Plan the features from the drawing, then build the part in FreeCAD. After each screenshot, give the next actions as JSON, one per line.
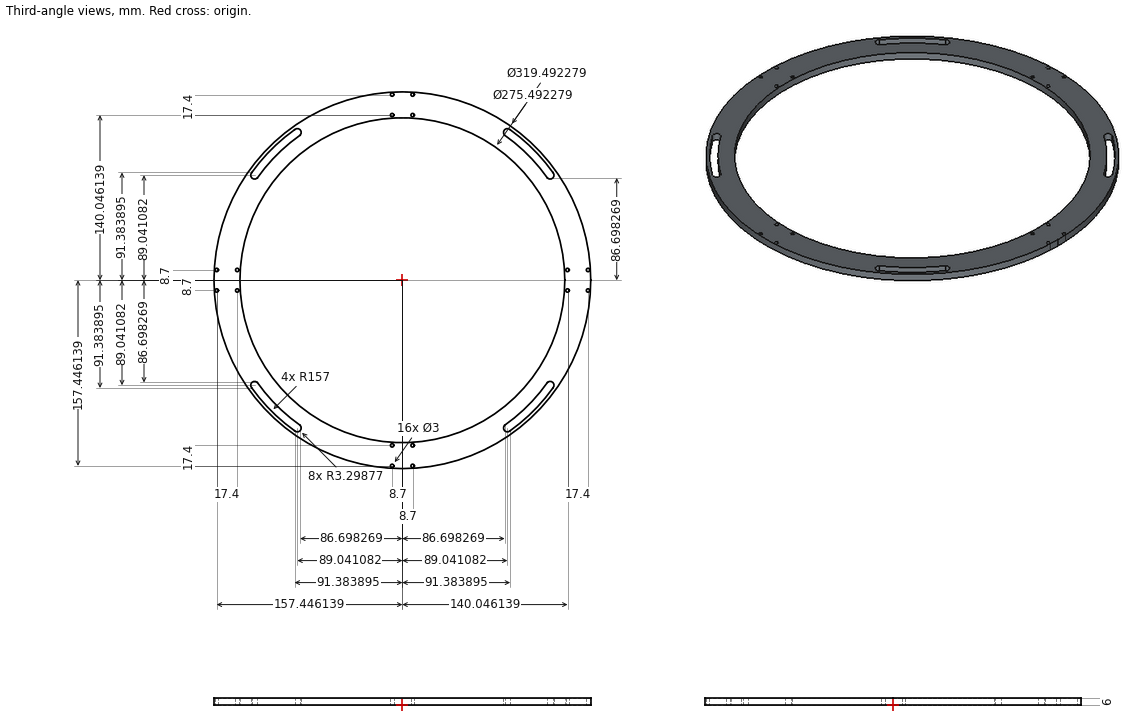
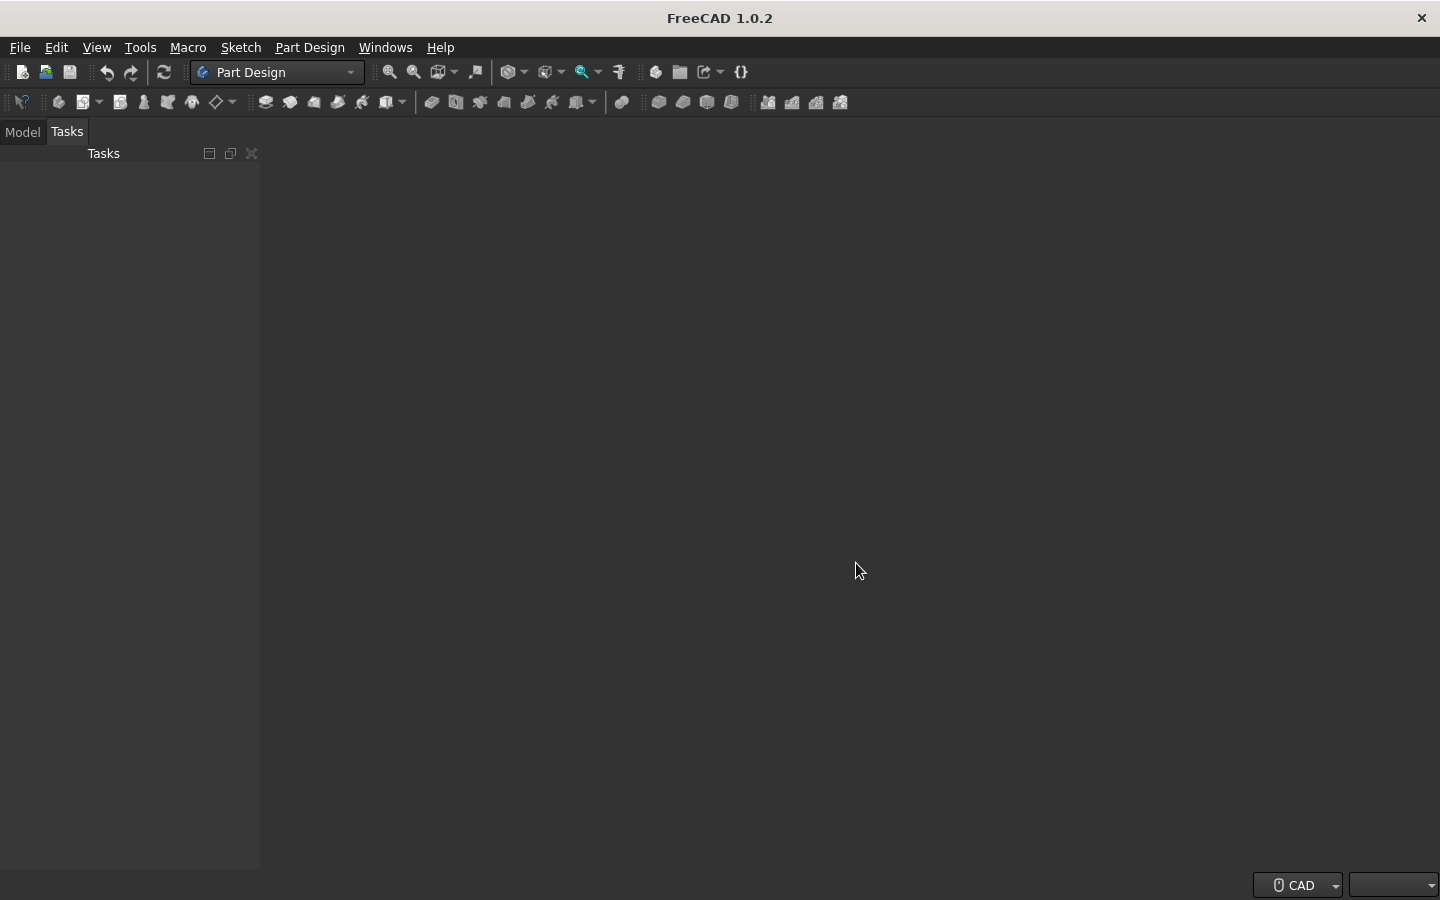
{"action": "key", "text": "ctrl+n"}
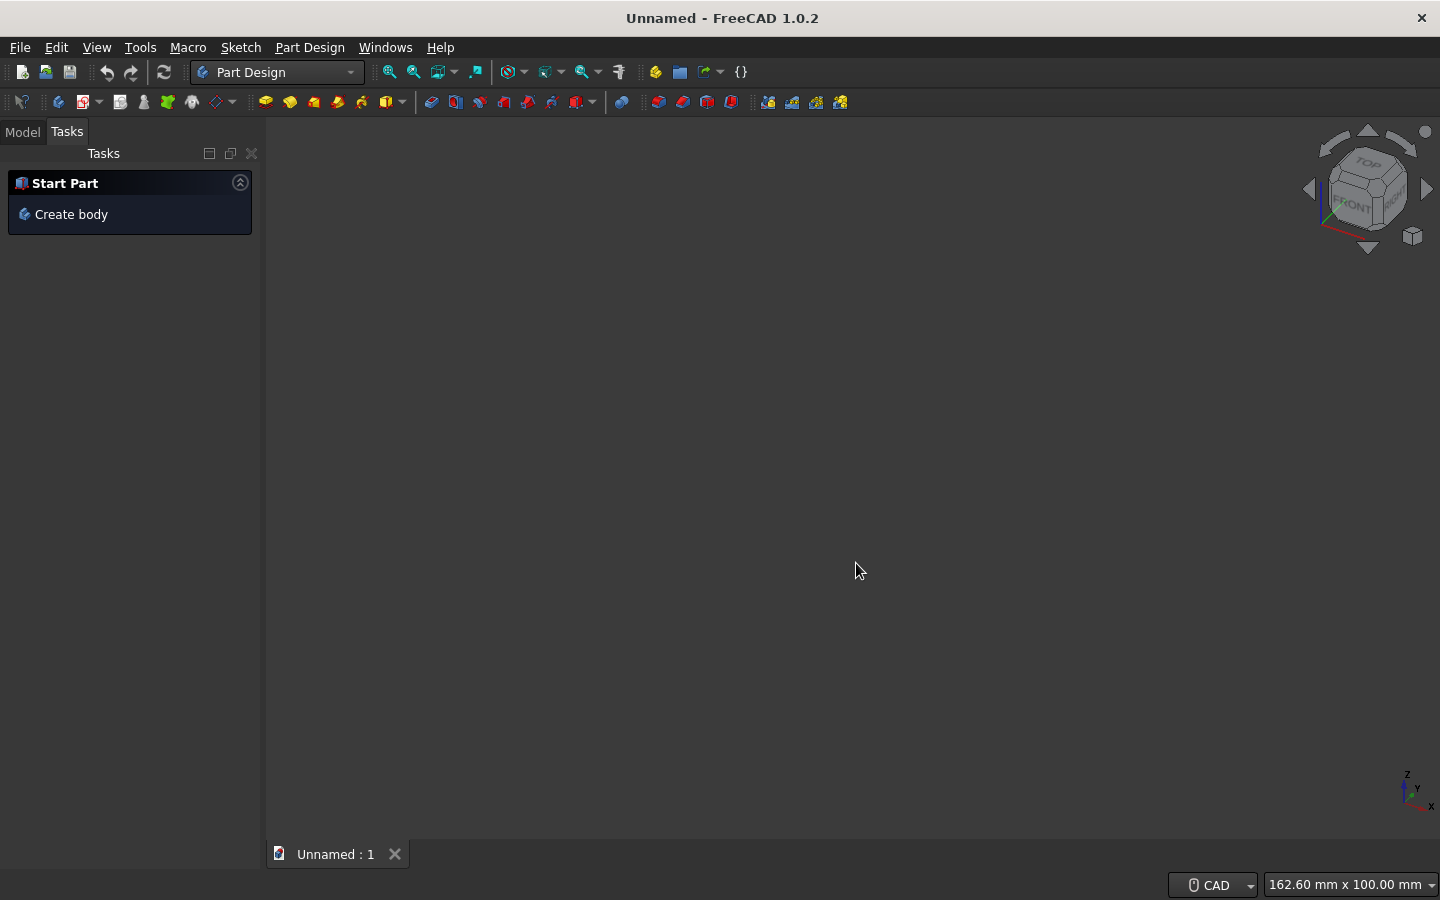
{"action": "left_click", "coordinate": [84, 102]}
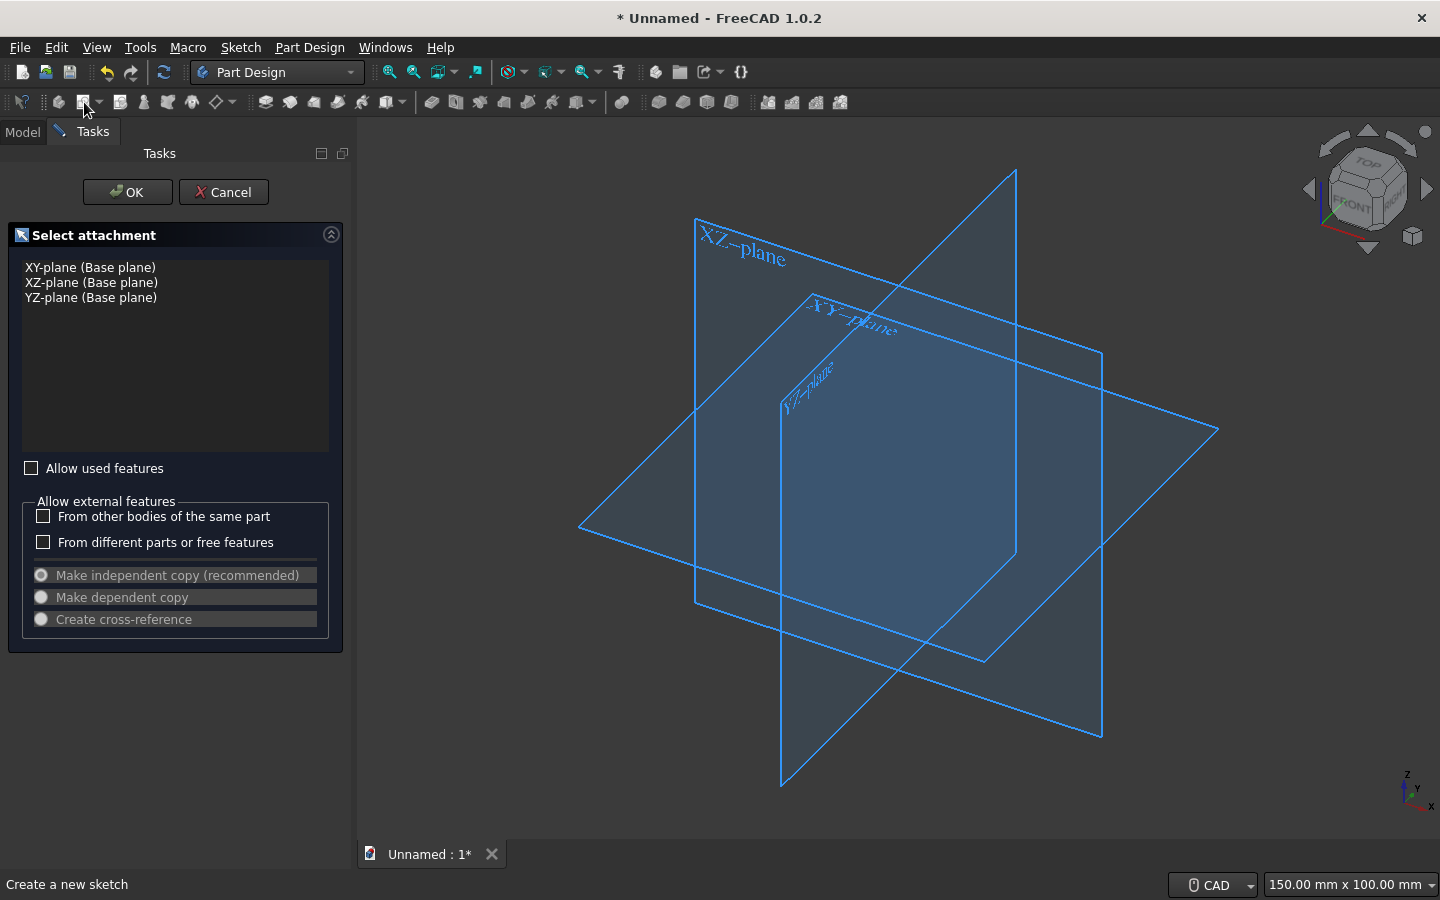
{"action": "left_click", "coordinate": [82, 268]}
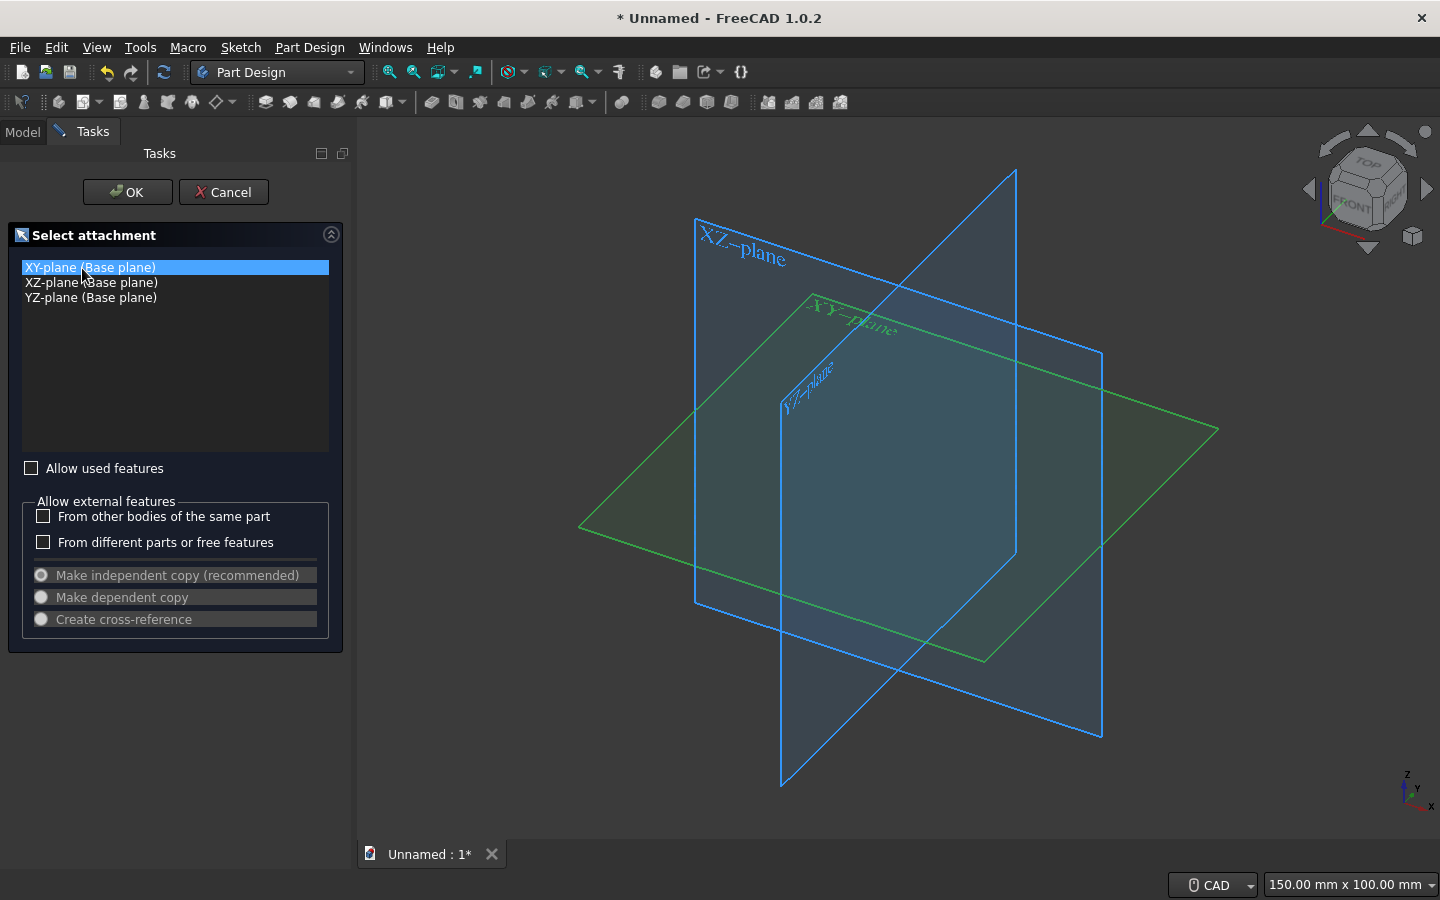
{"action": "left_click", "coordinate": [128, 192]}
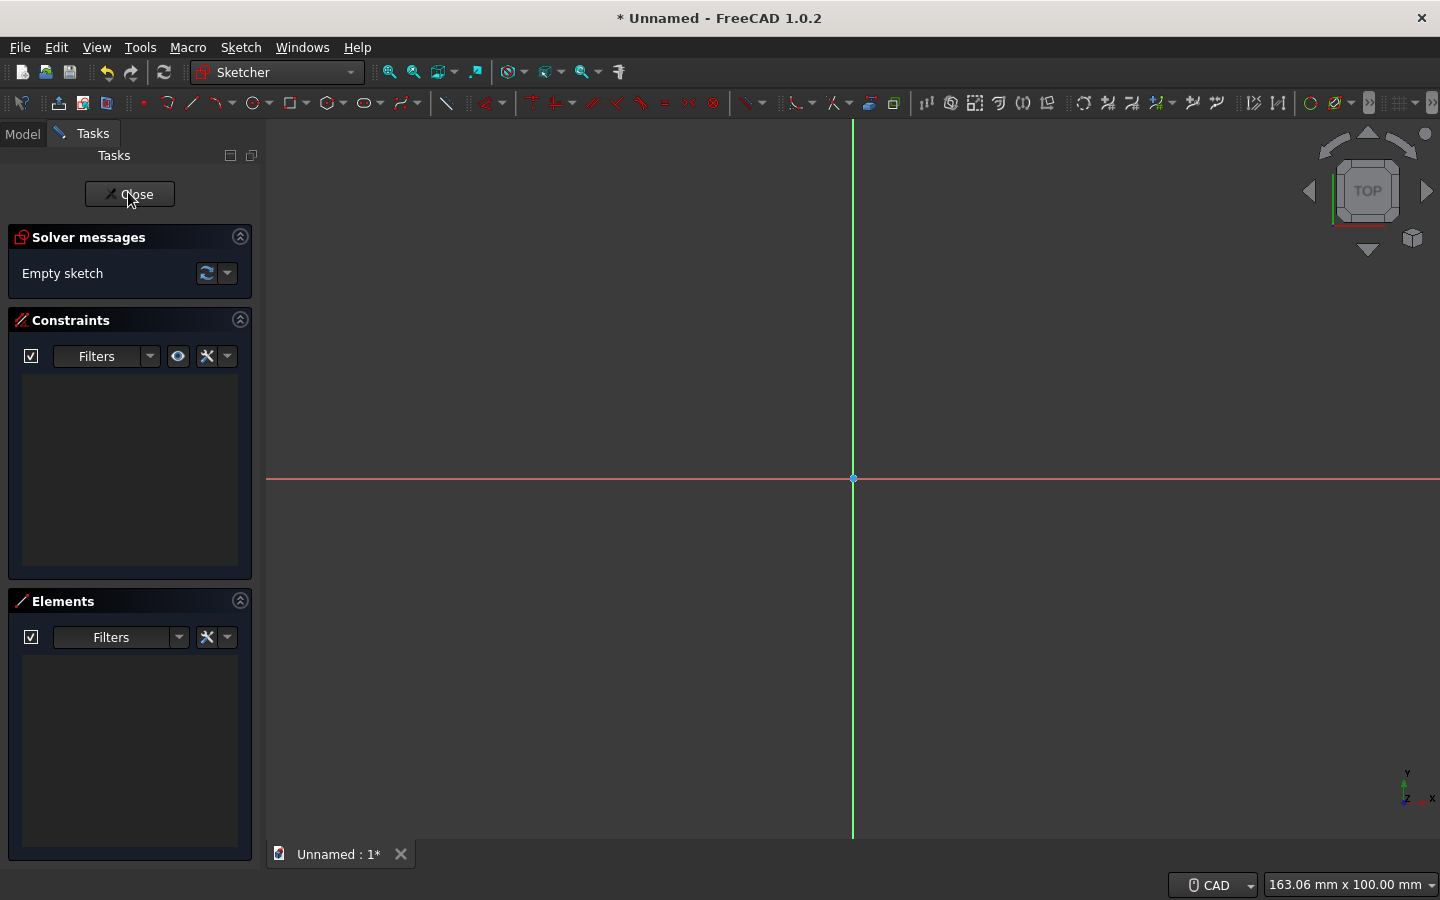
{"action": "scroll", "coordinate": [767, 479], "scroll_direction": "down", "scroll_amount": 8}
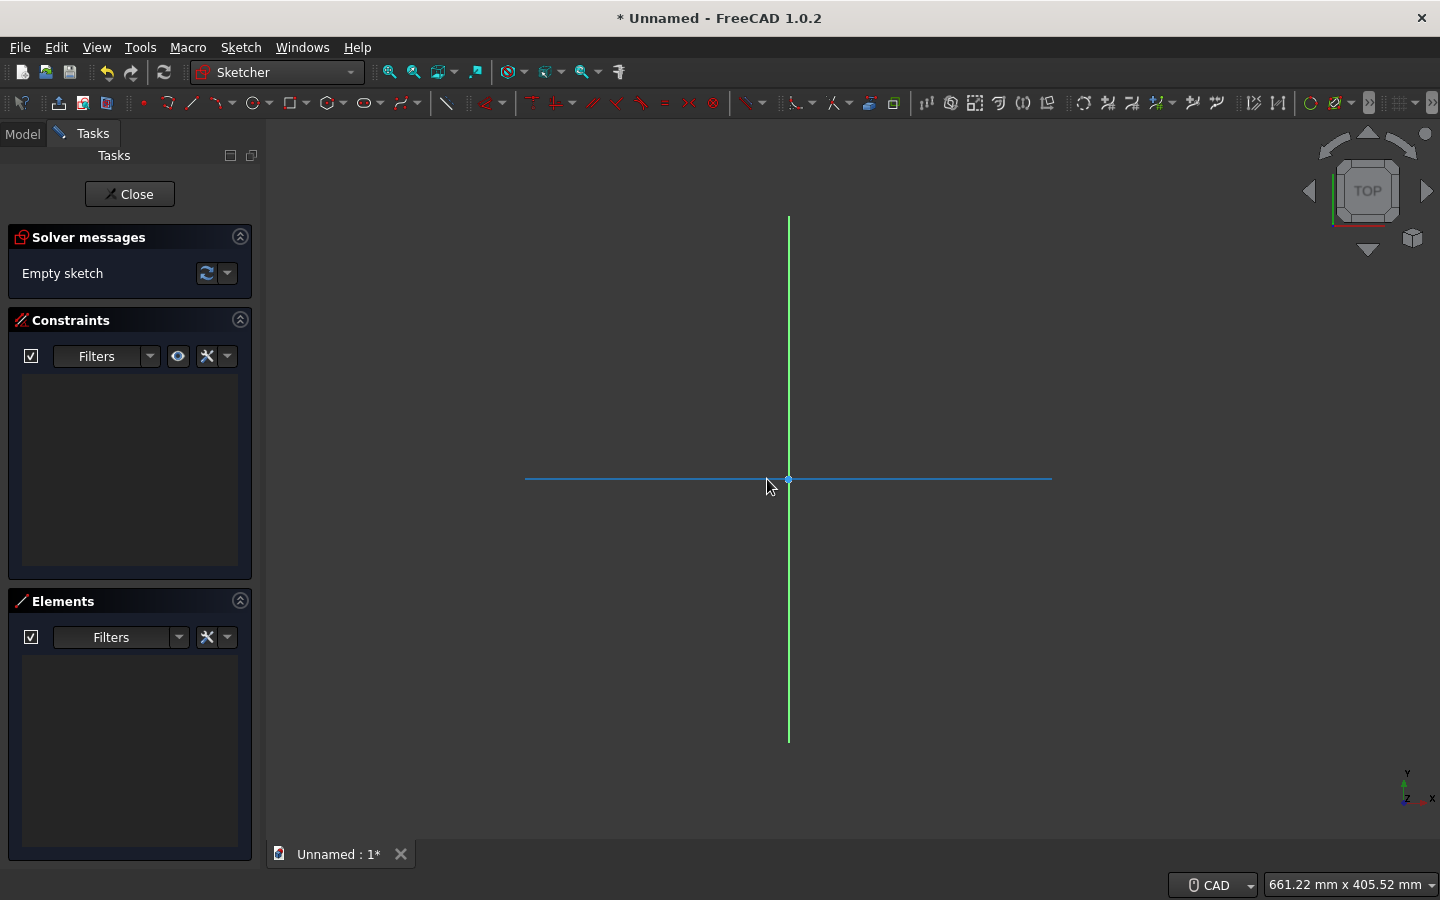
{"action": "key", "text": "g 3 a"}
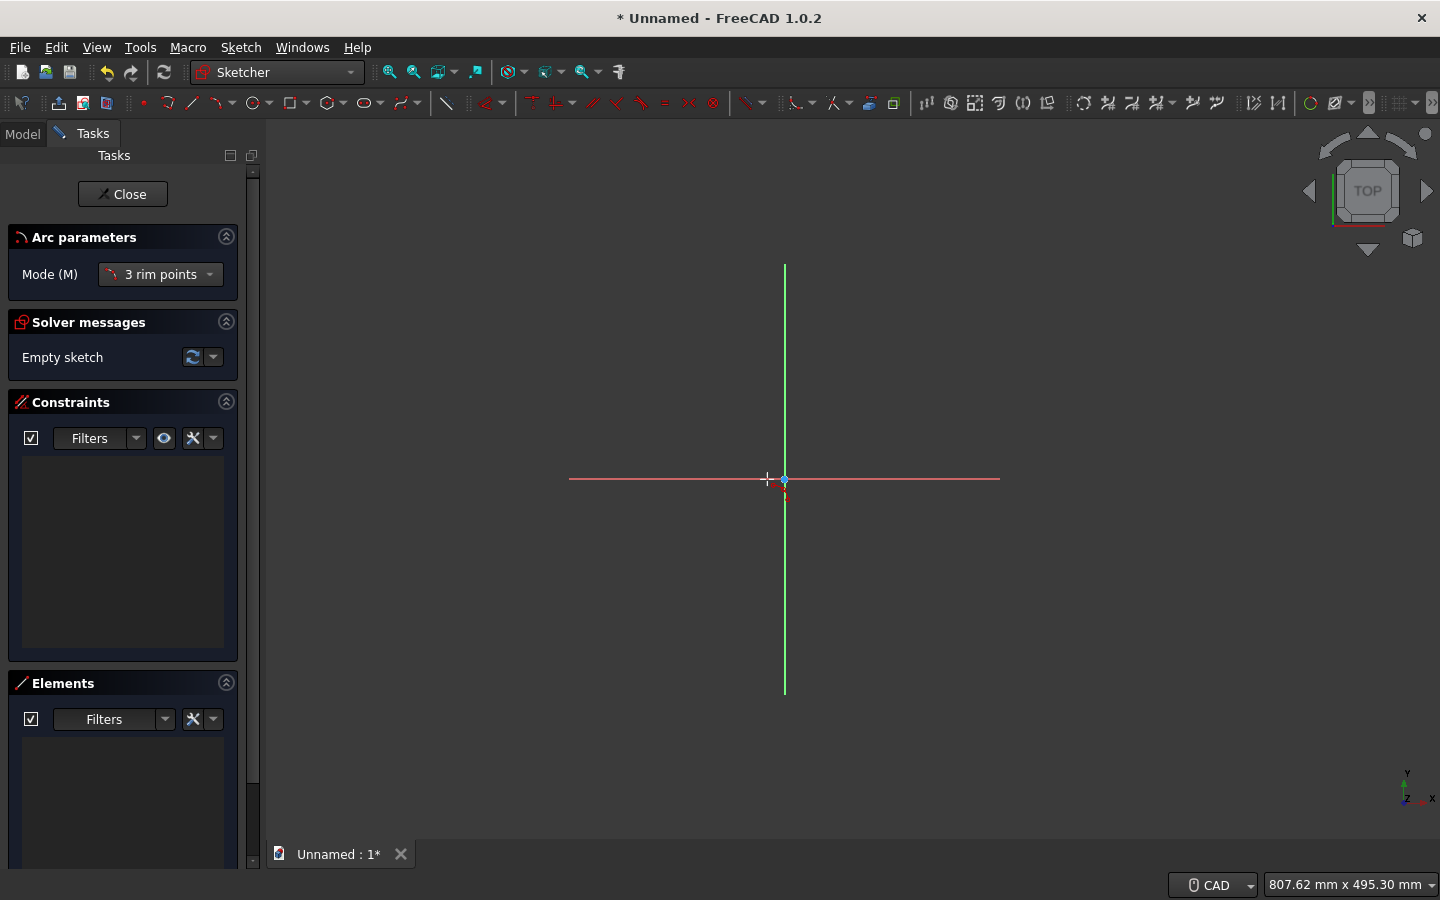
{"action": "left_click", "coordinate": [659, 658]}
{"action": "left_click", "coordinate": [652, 665]}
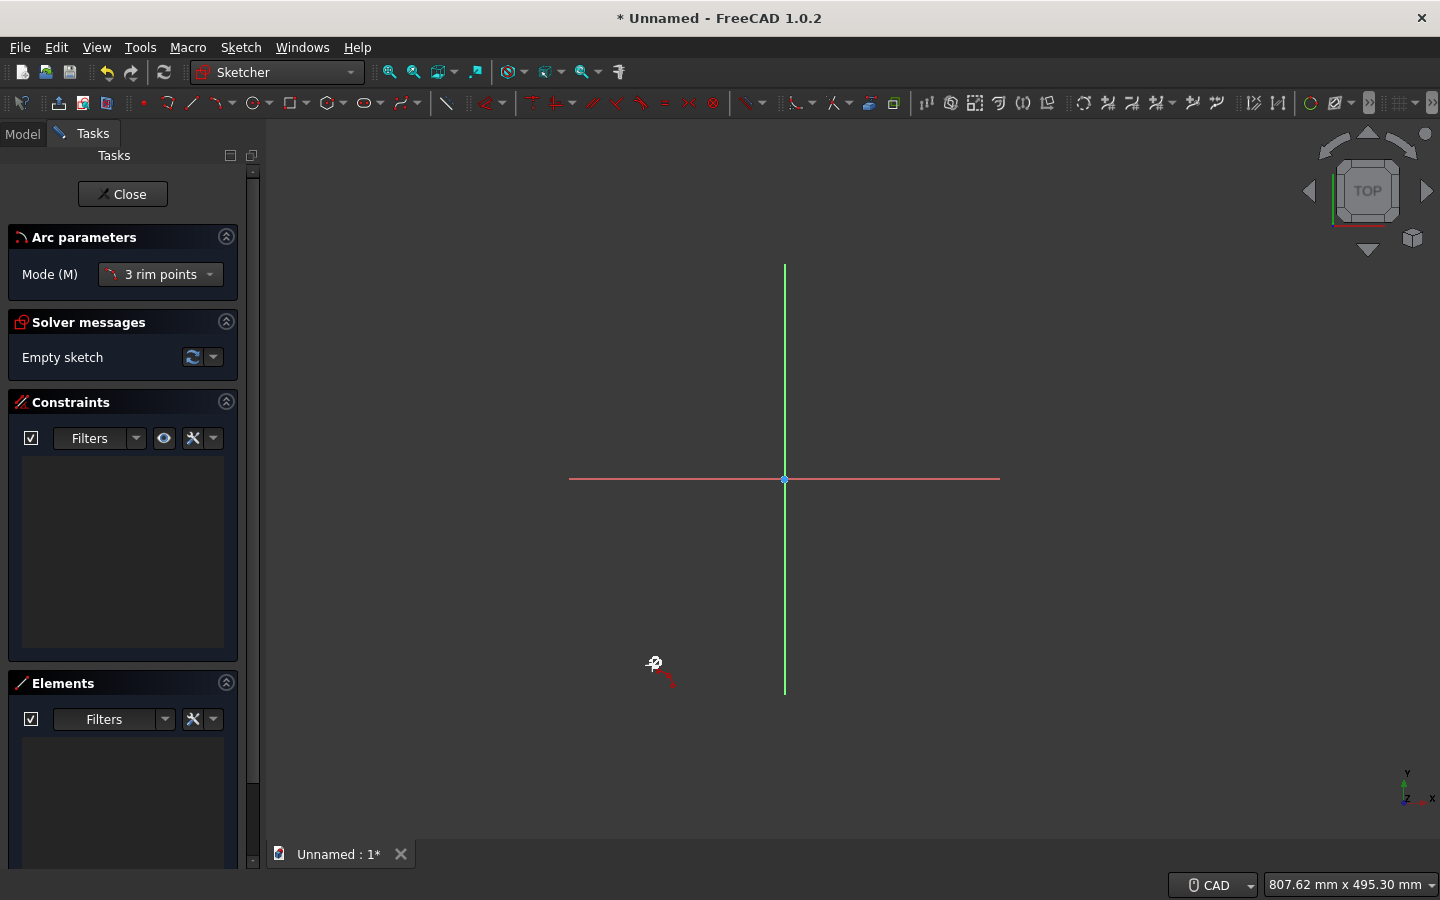
{"action": "scroll", "coordinate": [659, 665], "scroll_direction": "up", "scroll_amount": 6}